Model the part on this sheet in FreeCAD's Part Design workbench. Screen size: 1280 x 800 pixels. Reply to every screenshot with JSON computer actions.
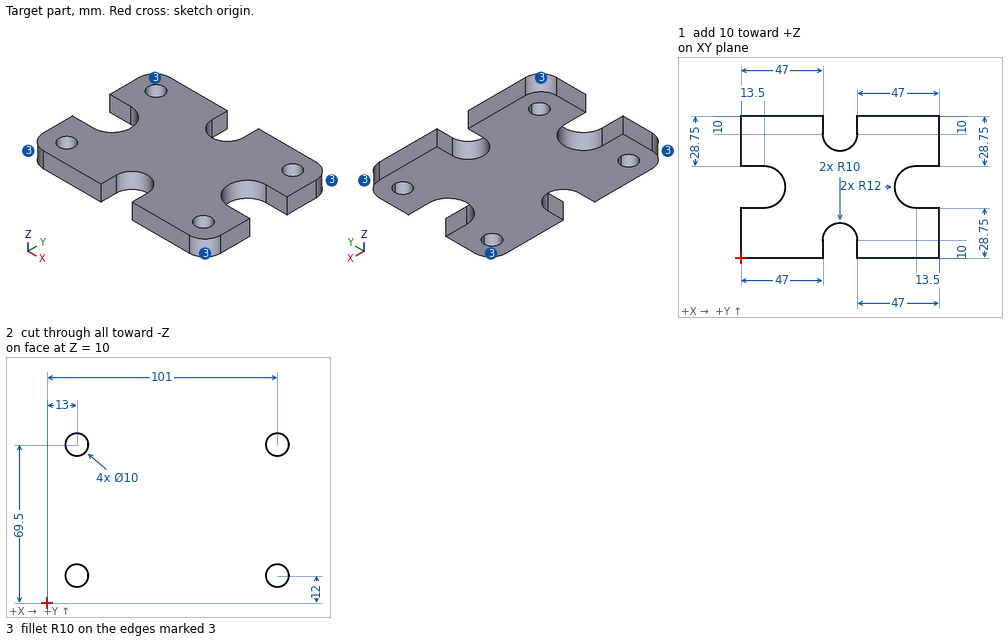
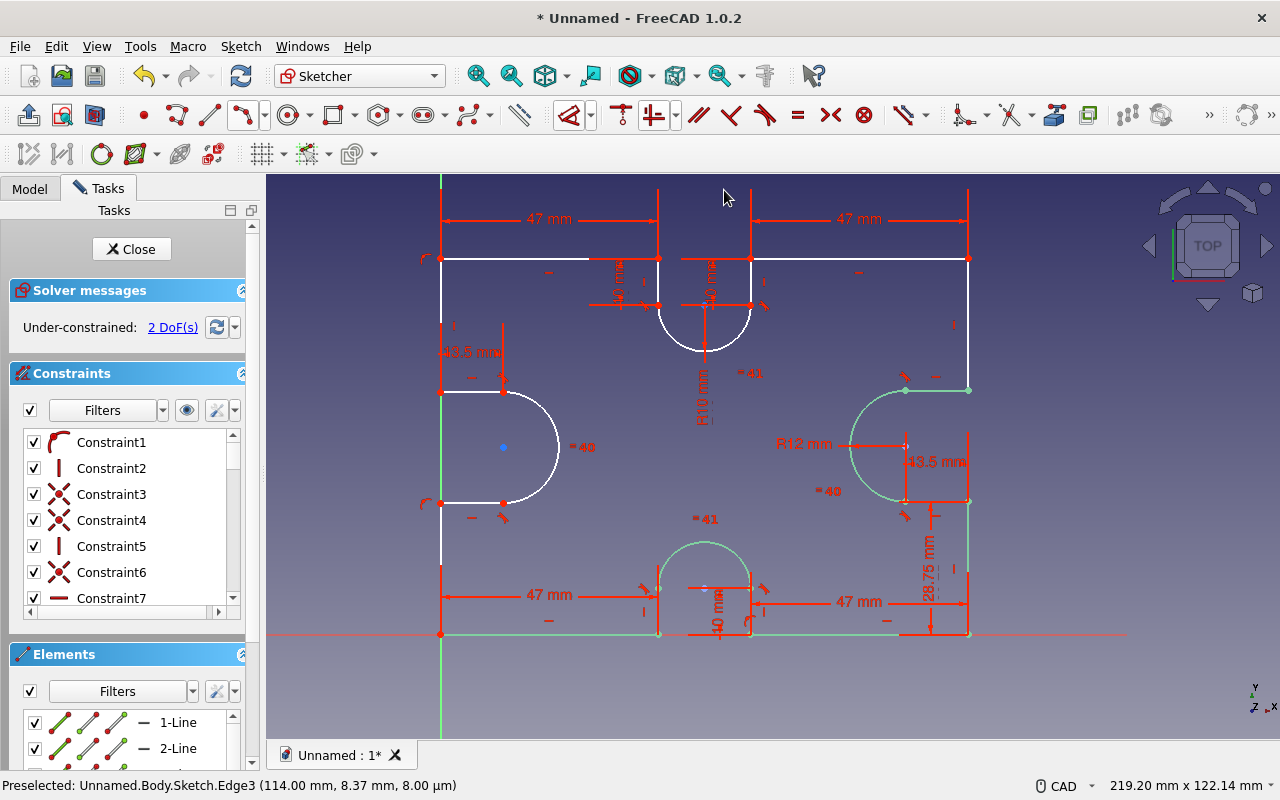
{"action": "left_click", "coordinate": [968, 351]}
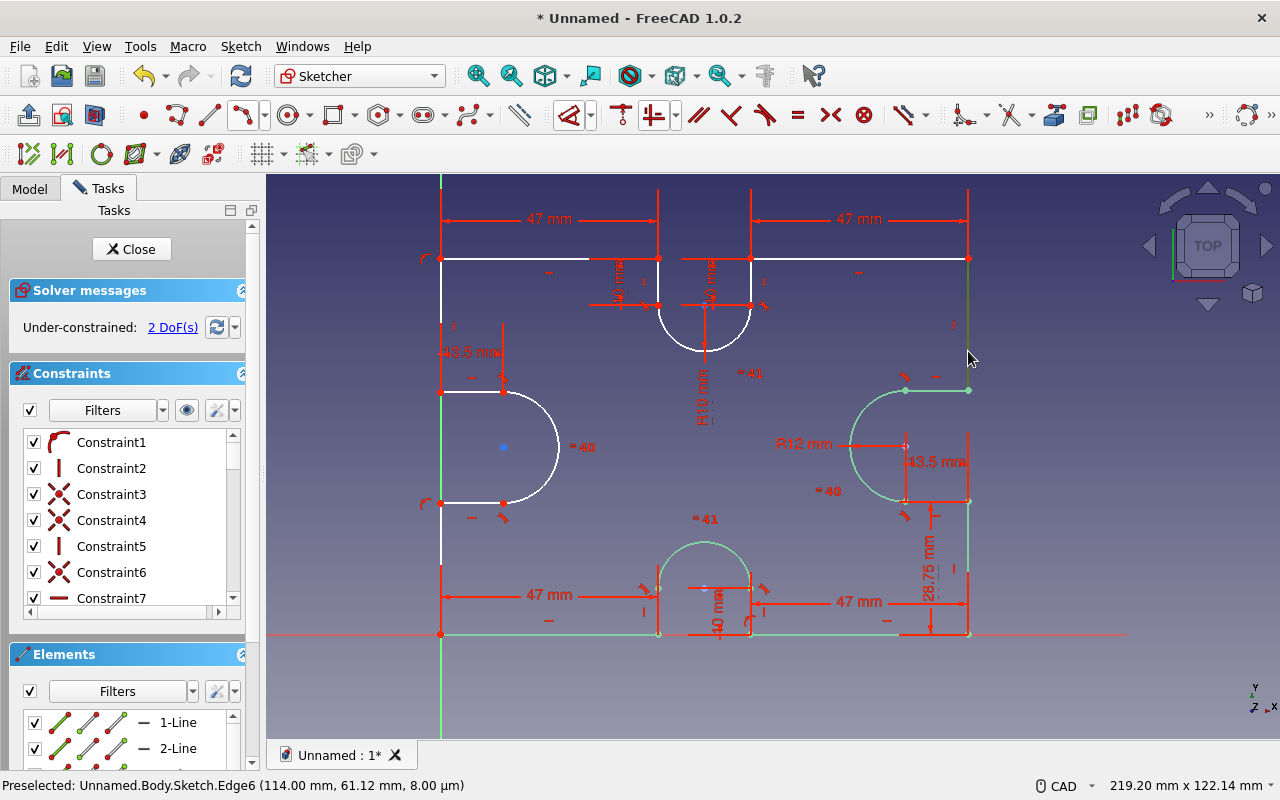
{"action": "key", "text": "i"}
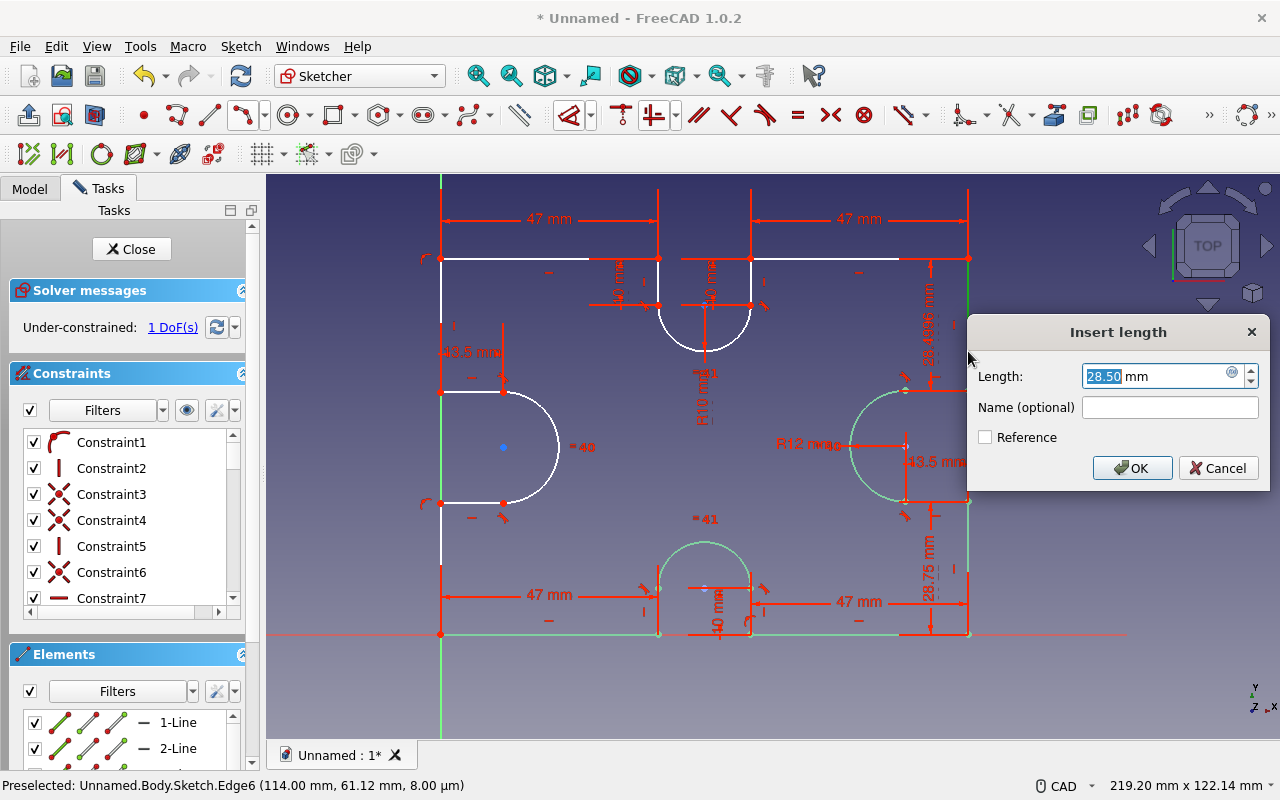
{"action": "type", "text": "28.75"}
{"action": "key", "text": "Return"}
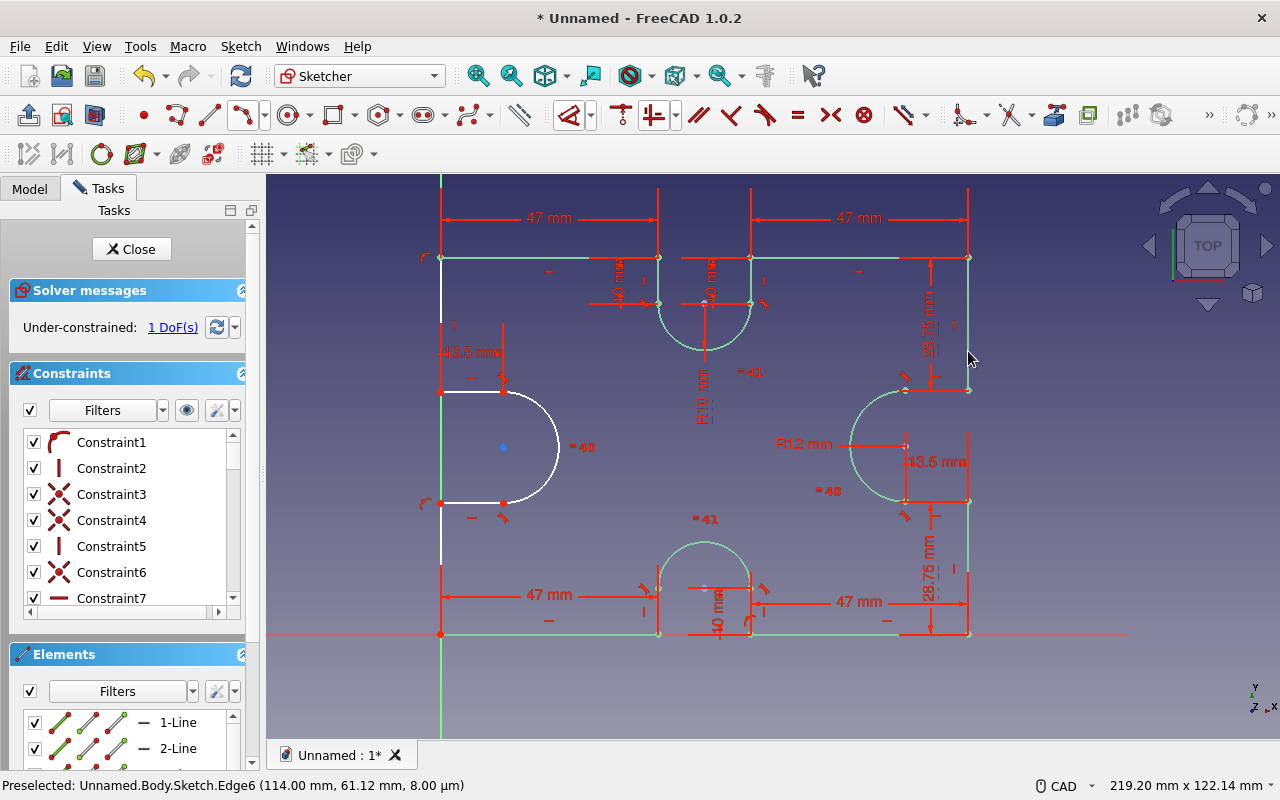
{"action": "left_click", "coordinate": [441, 298]}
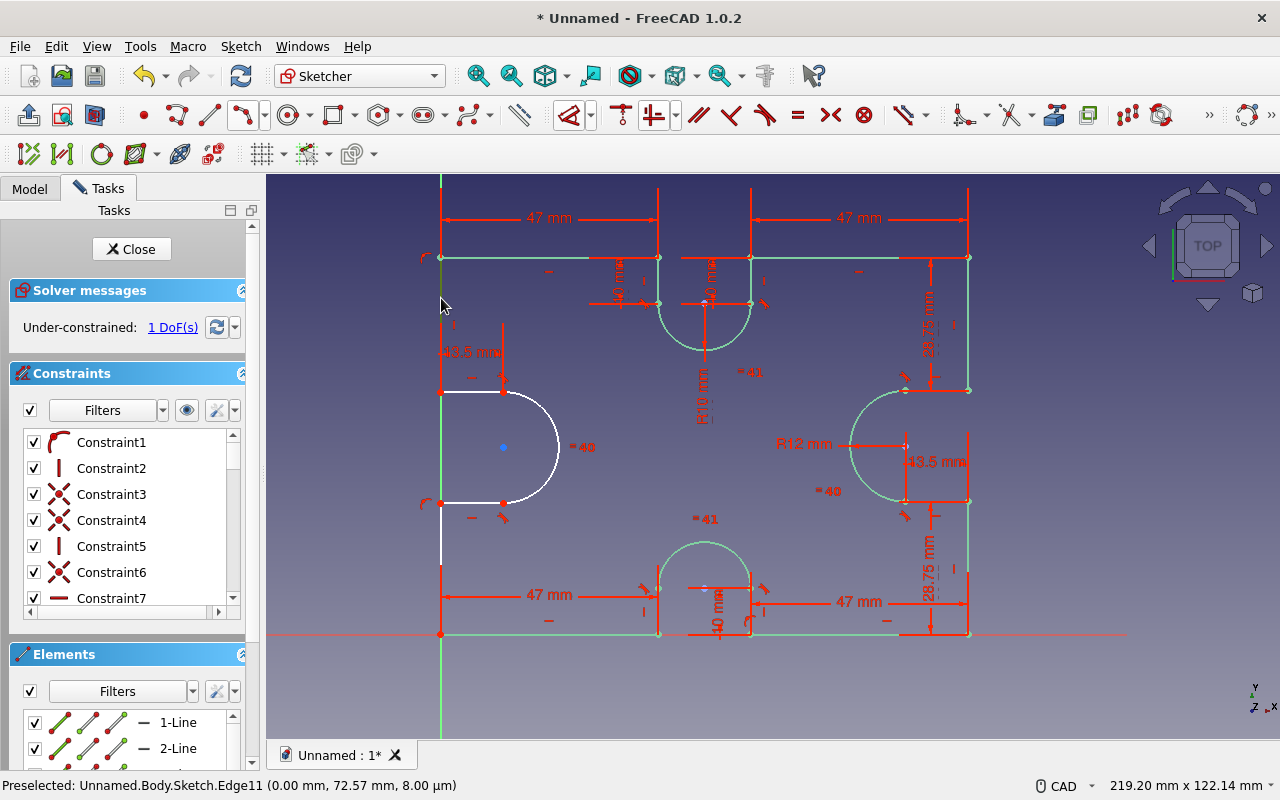
{"action": "left_click", "coordinate": [590, 116]}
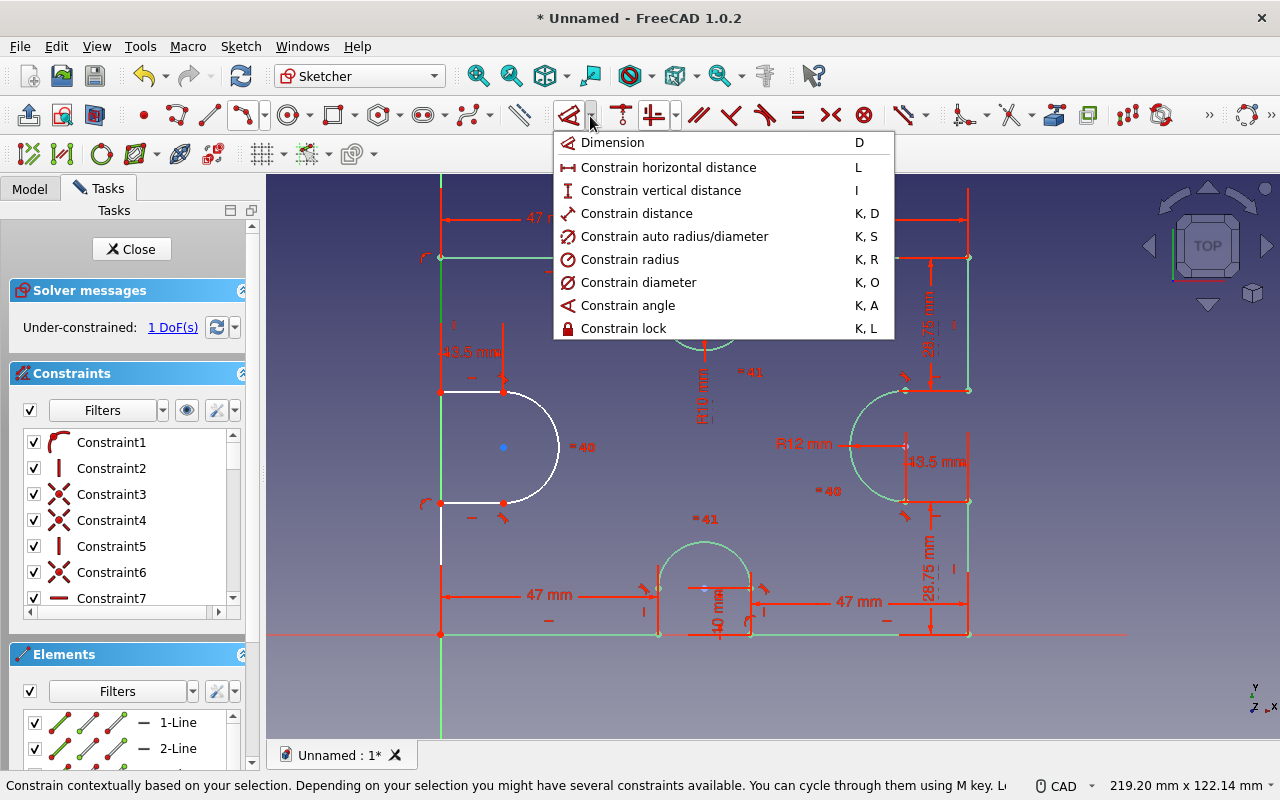
{"action": "left_click", "coordinate": [724, 190]}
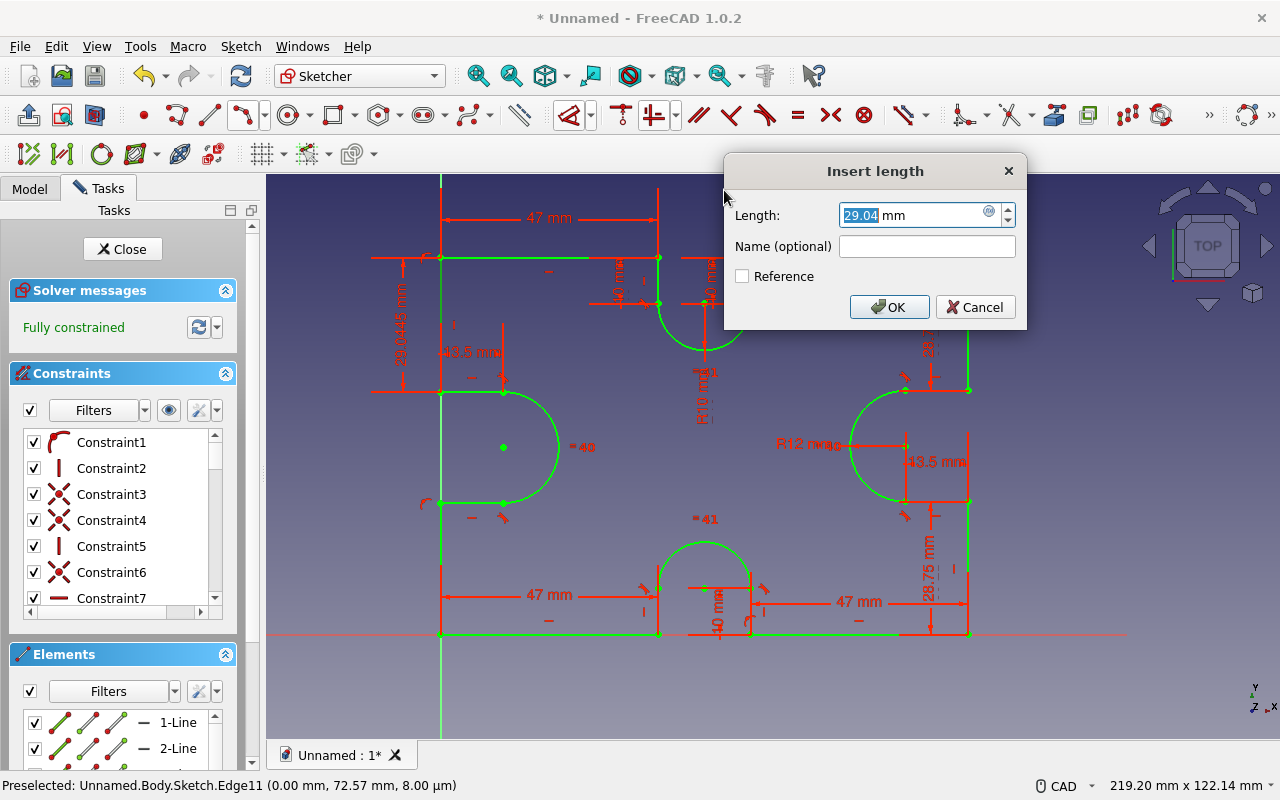
{"action": "type", "text": "28.75"}
{"action": "key", "text": "Return"}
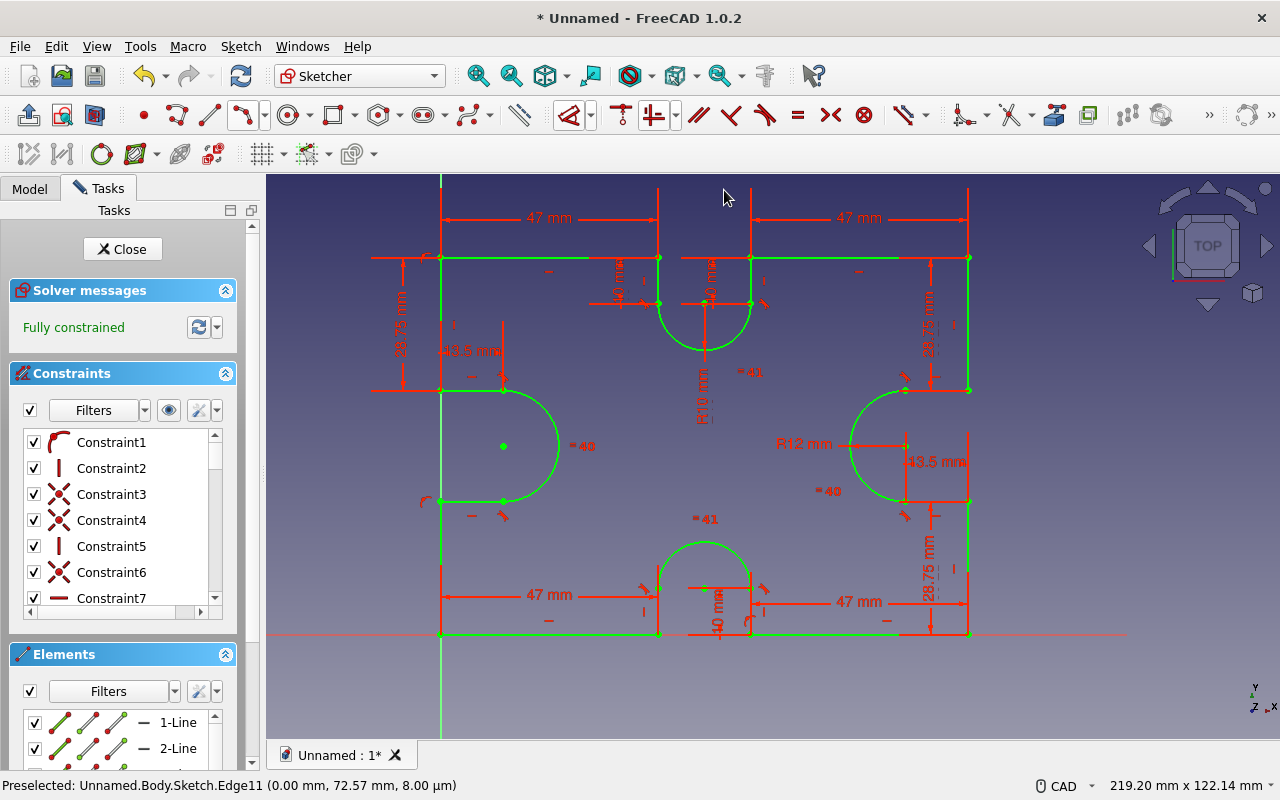
{"action": "left_click", "coordinate": [123, 249]}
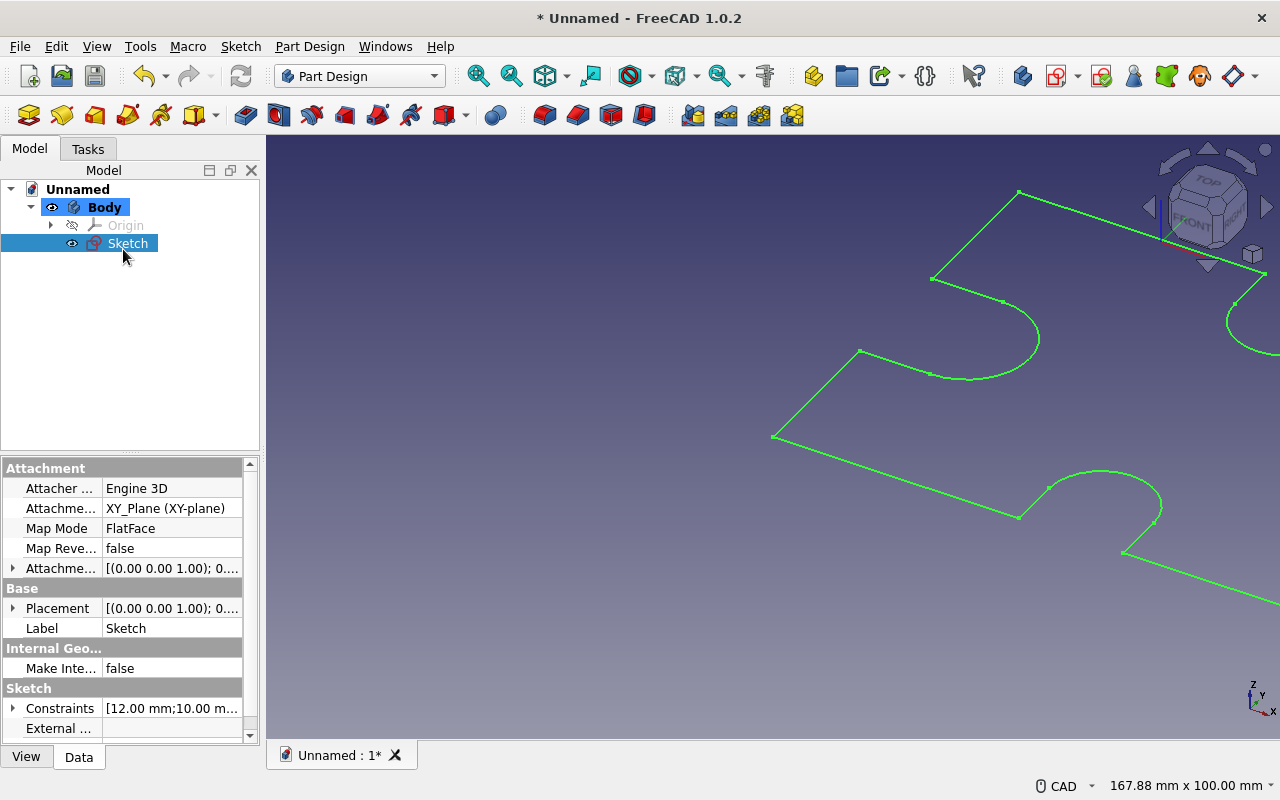
{"action": "left_click", "coordinate": [29, 116]}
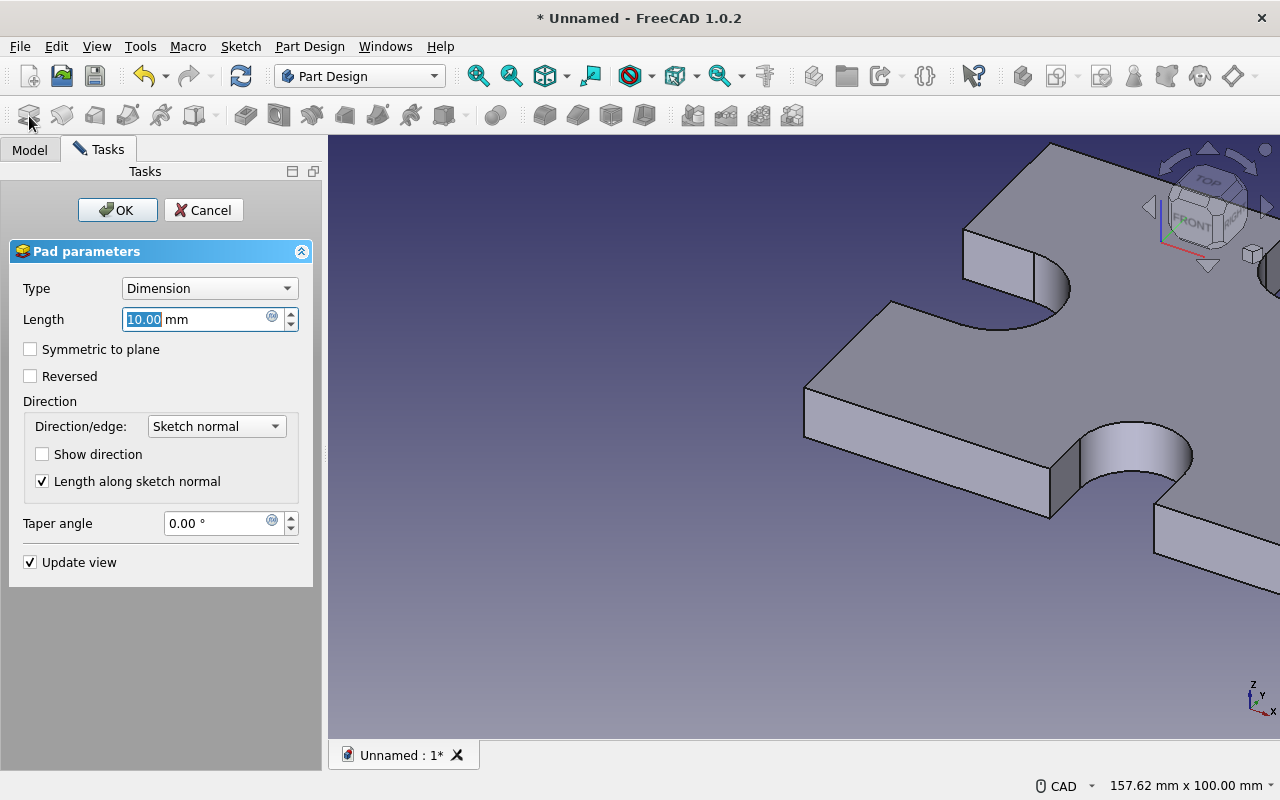
{"action": "type", "text": "10"}
{"action": "key", "text": "Tab"}